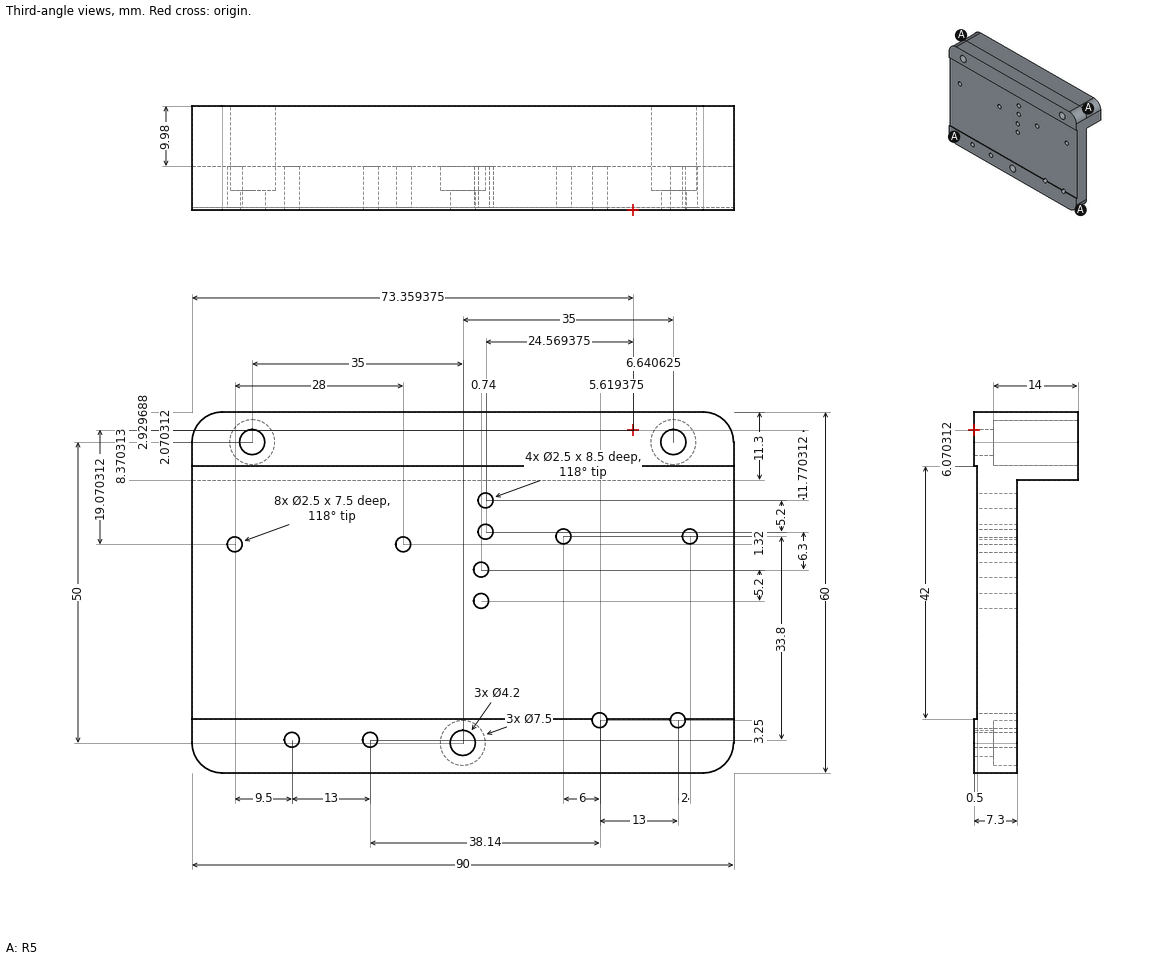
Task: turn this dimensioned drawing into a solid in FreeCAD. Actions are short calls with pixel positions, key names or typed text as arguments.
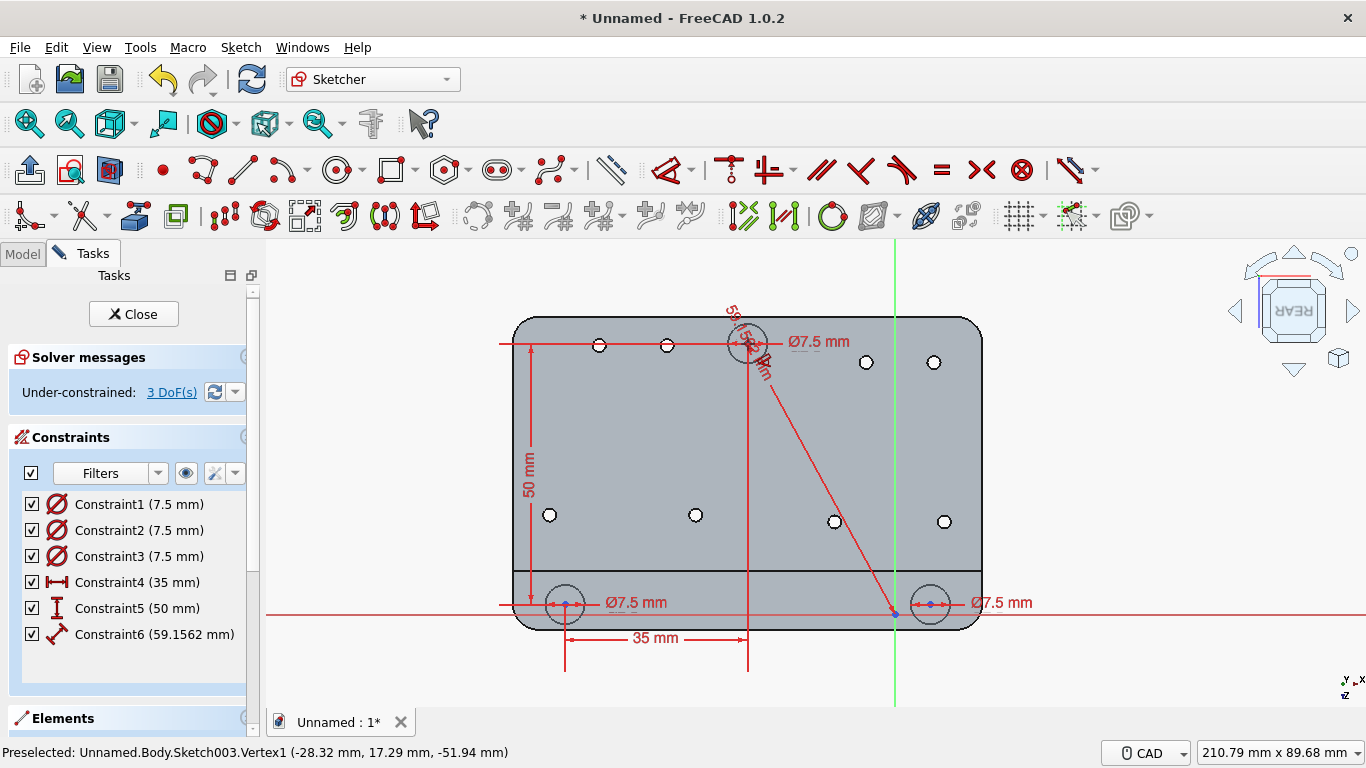
click(930, 605)
click(839, 639)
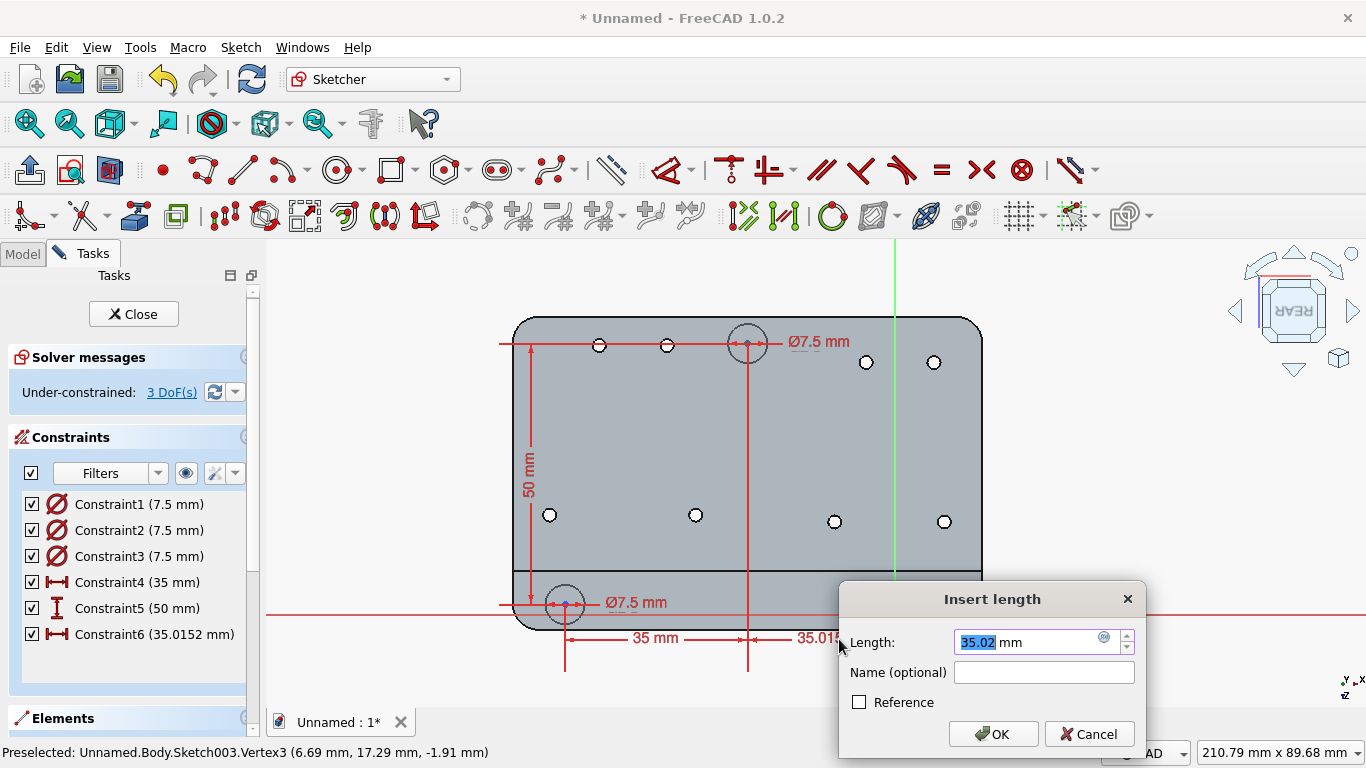
text(35)
key(Return)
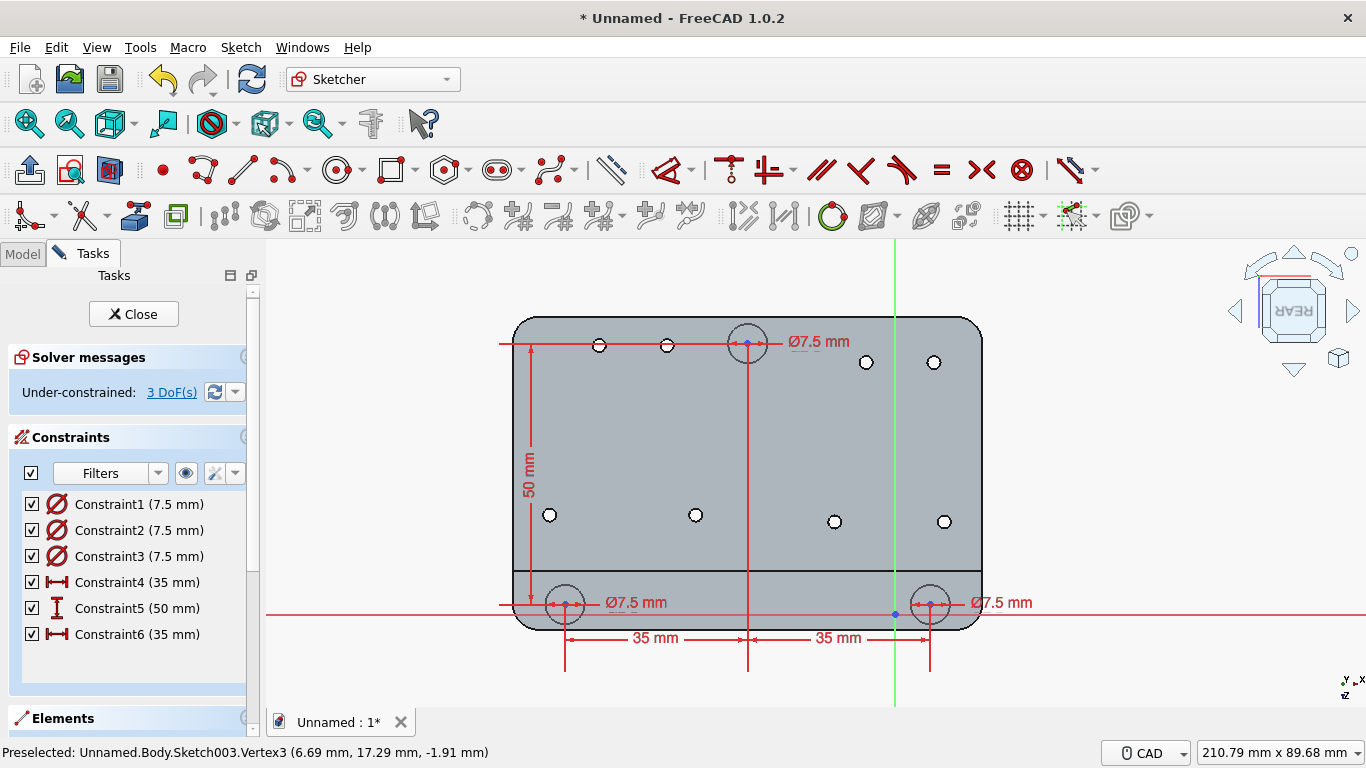
click(748, 344)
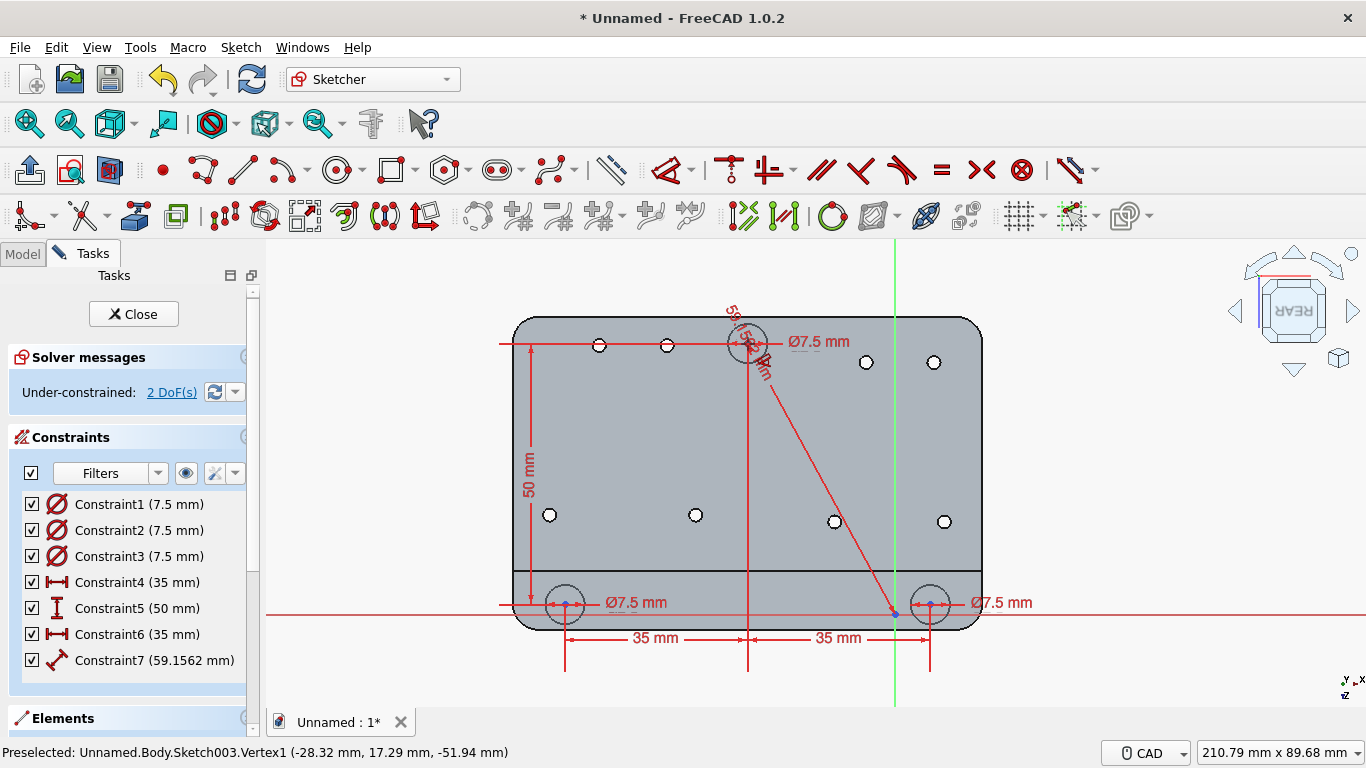
click(930, 605)
click(964, 474)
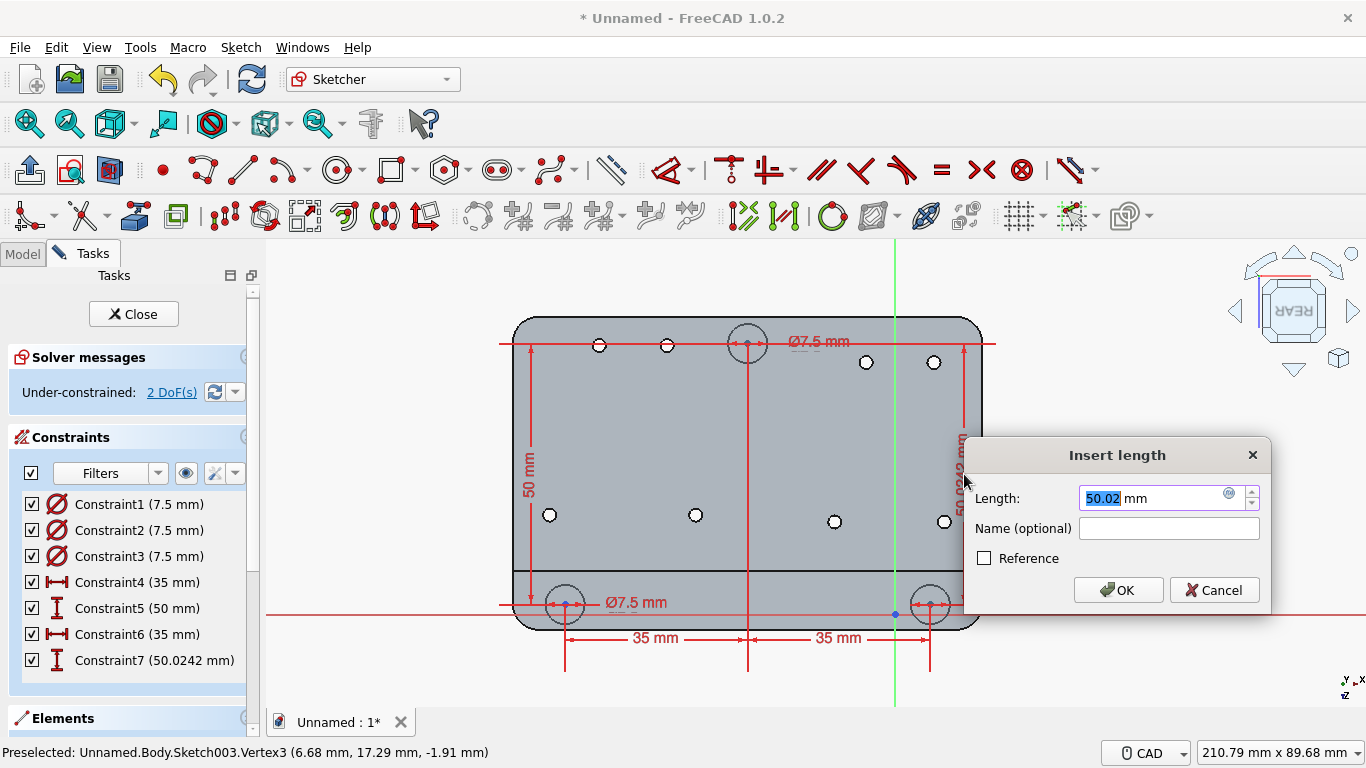
text(50)
key(Return)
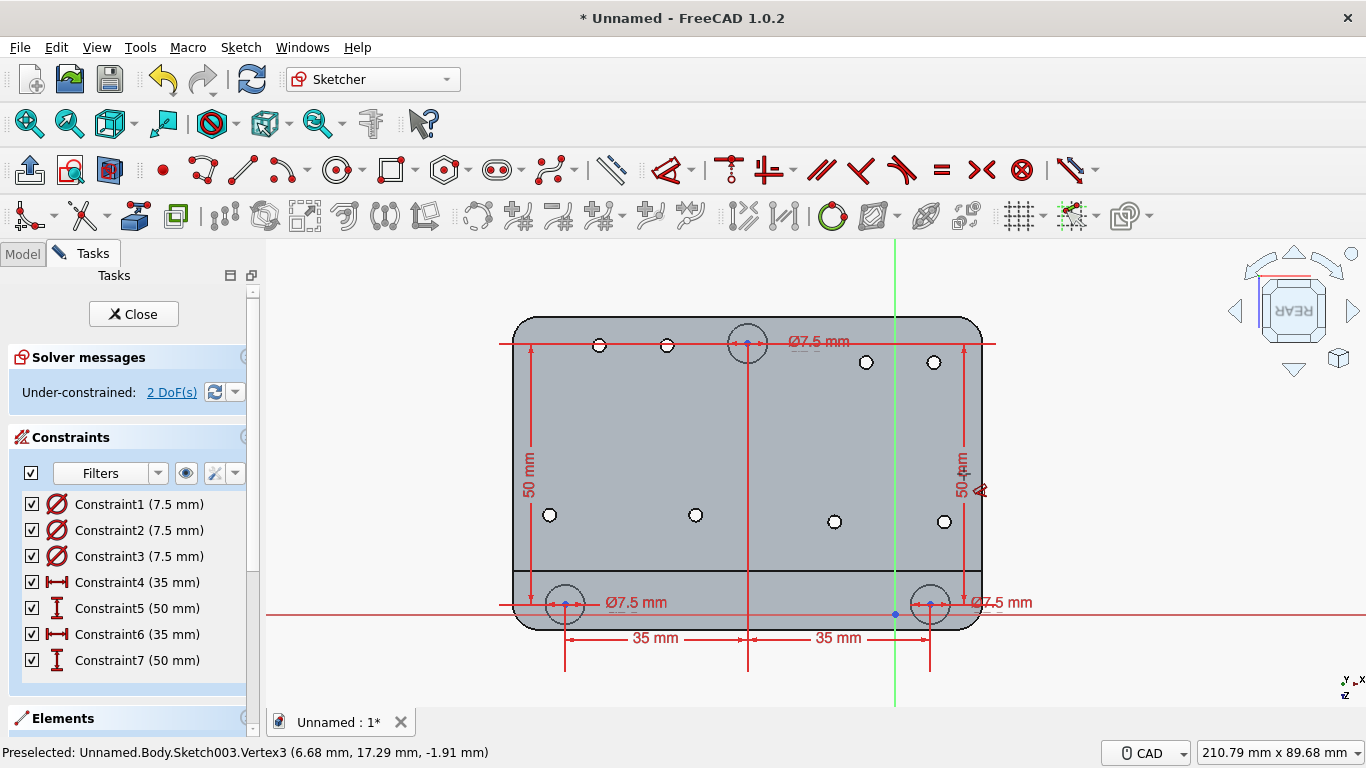
scroll(565, 605, up, 7)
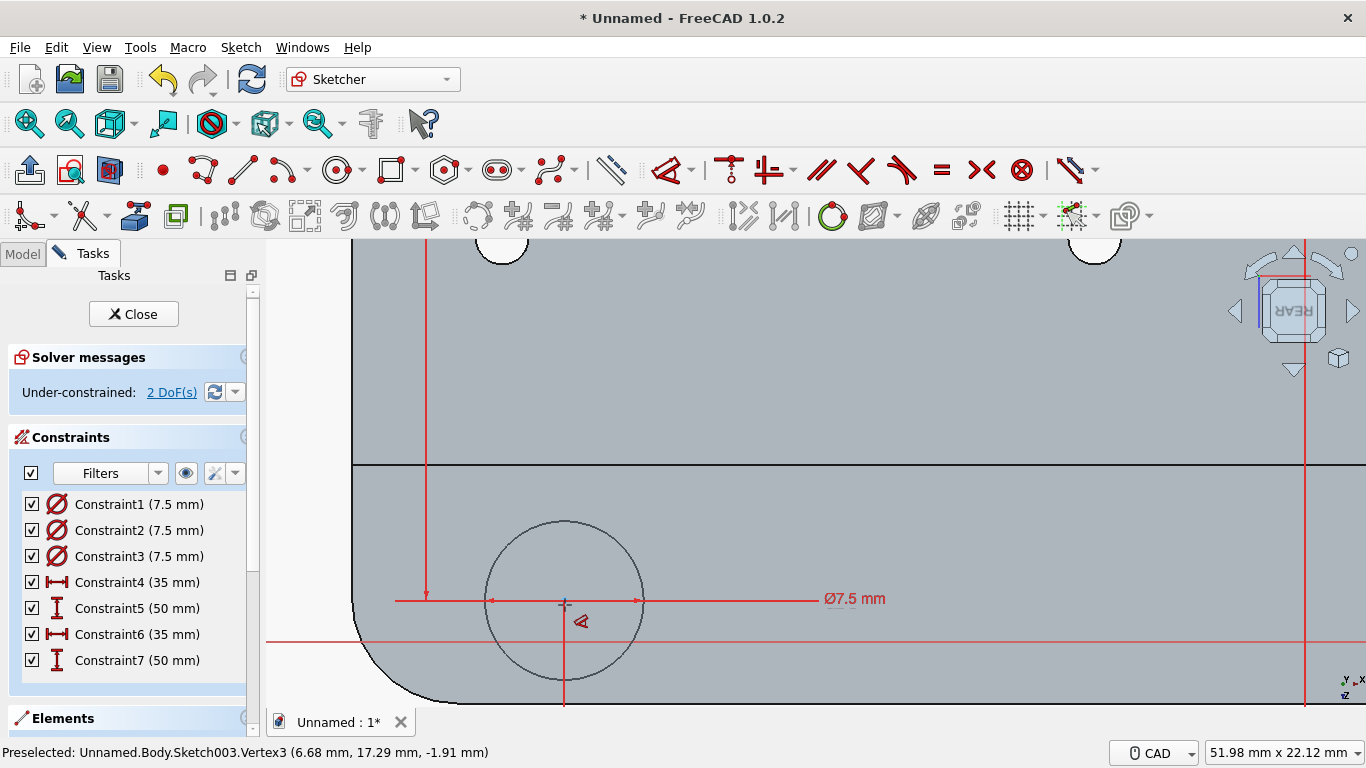
click(564, 601)
click(530, 621)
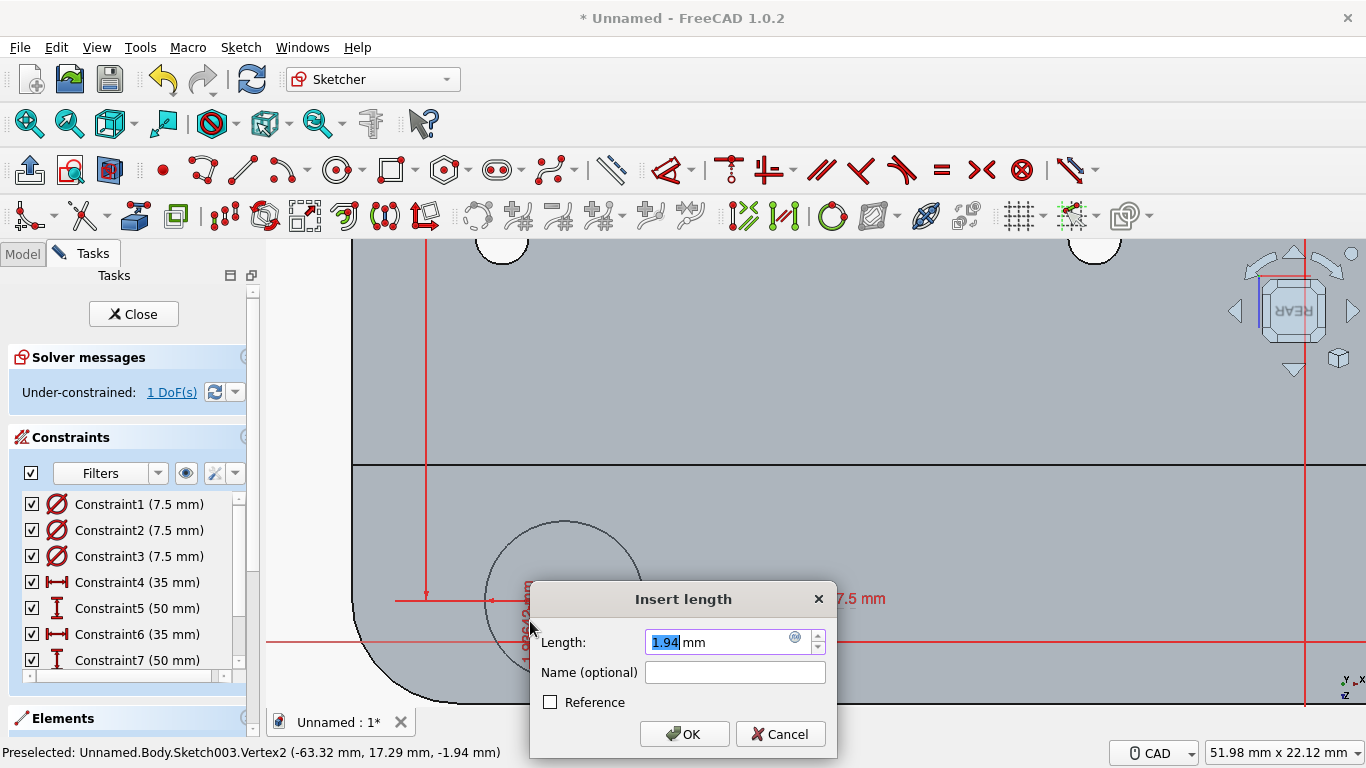
text(2.070312)
key(Return)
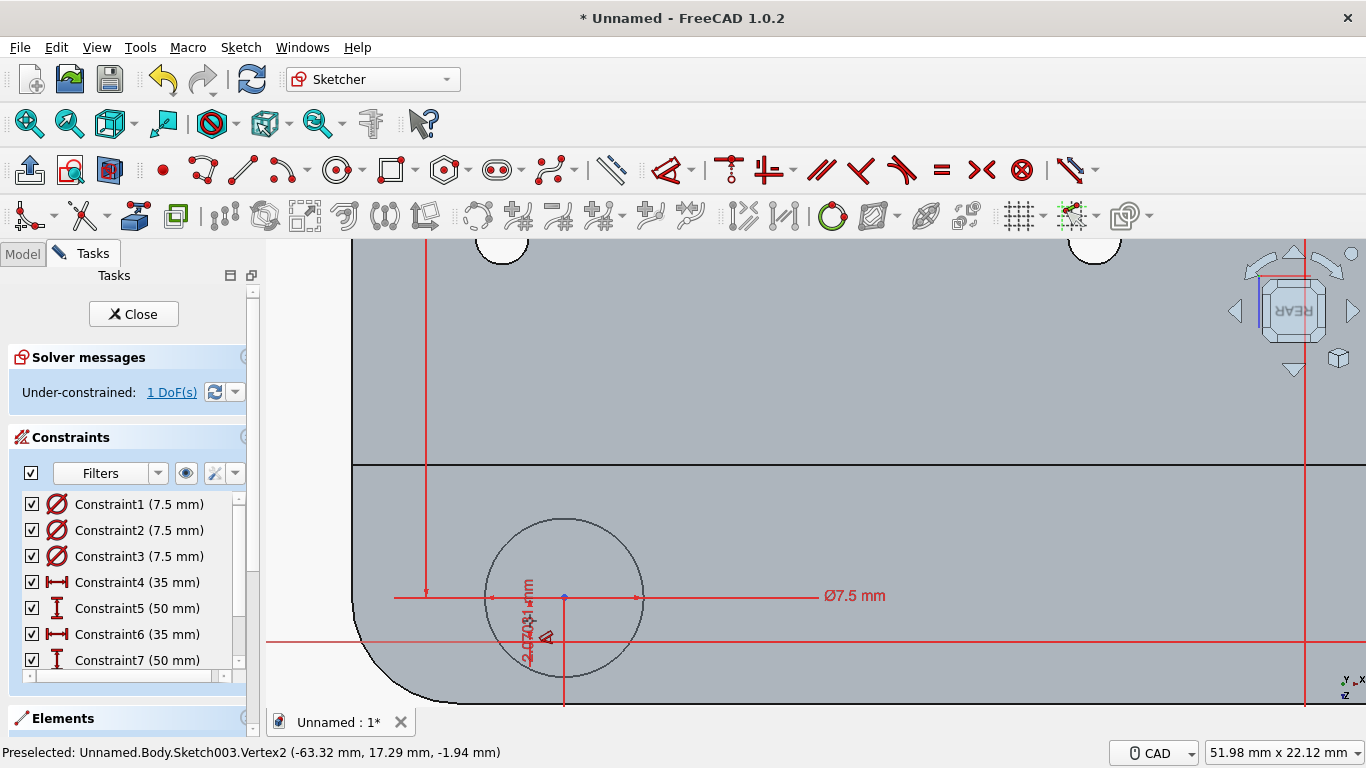
scroll(565, 605, down, 7)